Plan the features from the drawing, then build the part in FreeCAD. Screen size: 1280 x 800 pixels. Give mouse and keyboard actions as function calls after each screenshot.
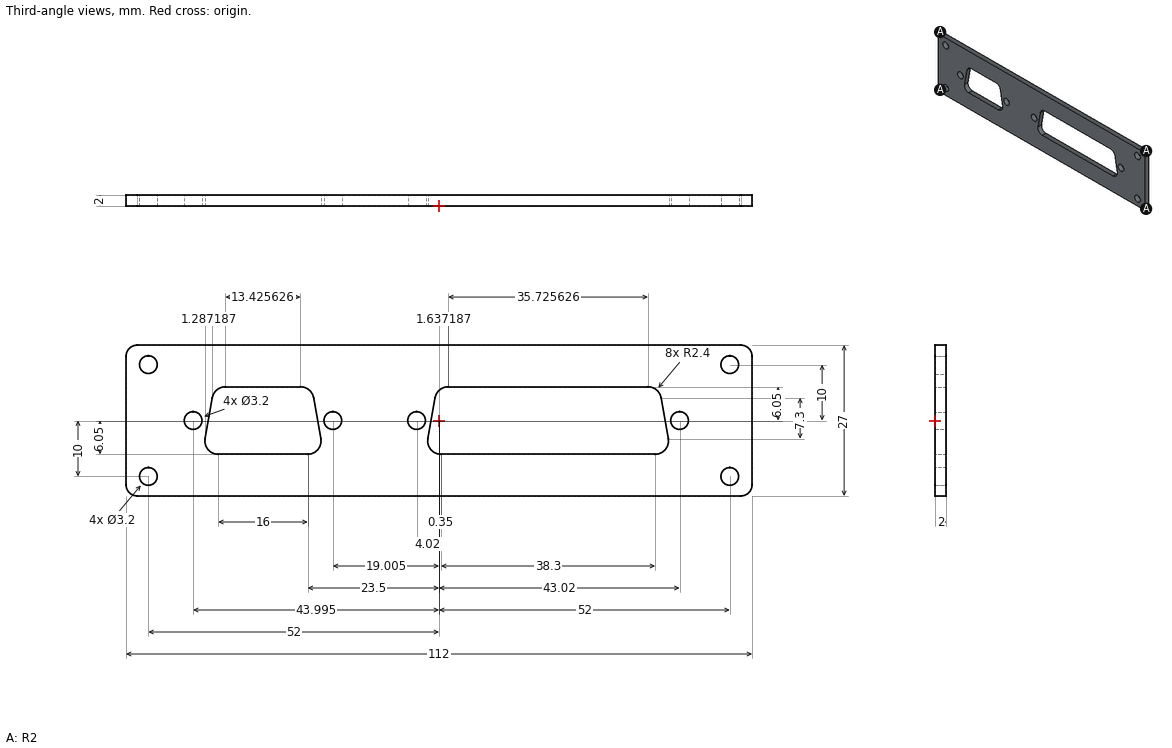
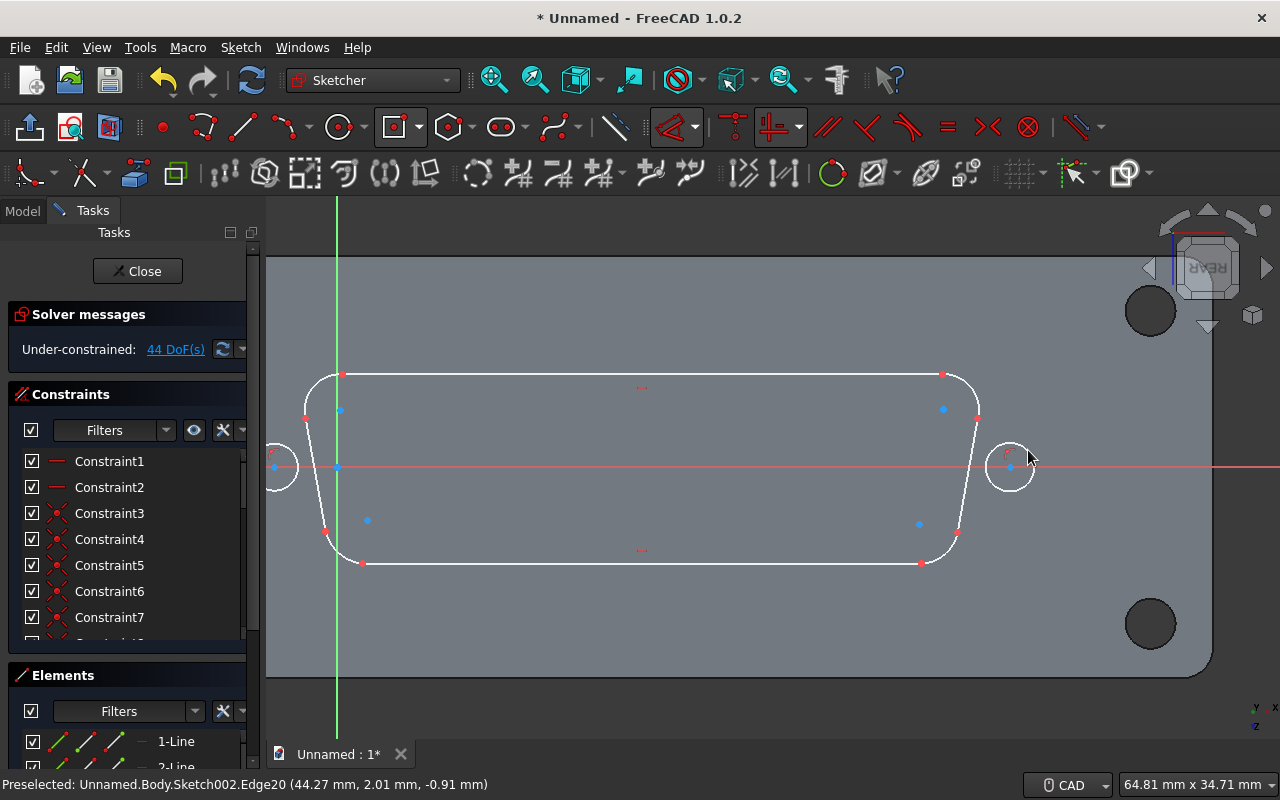
click(530, 564)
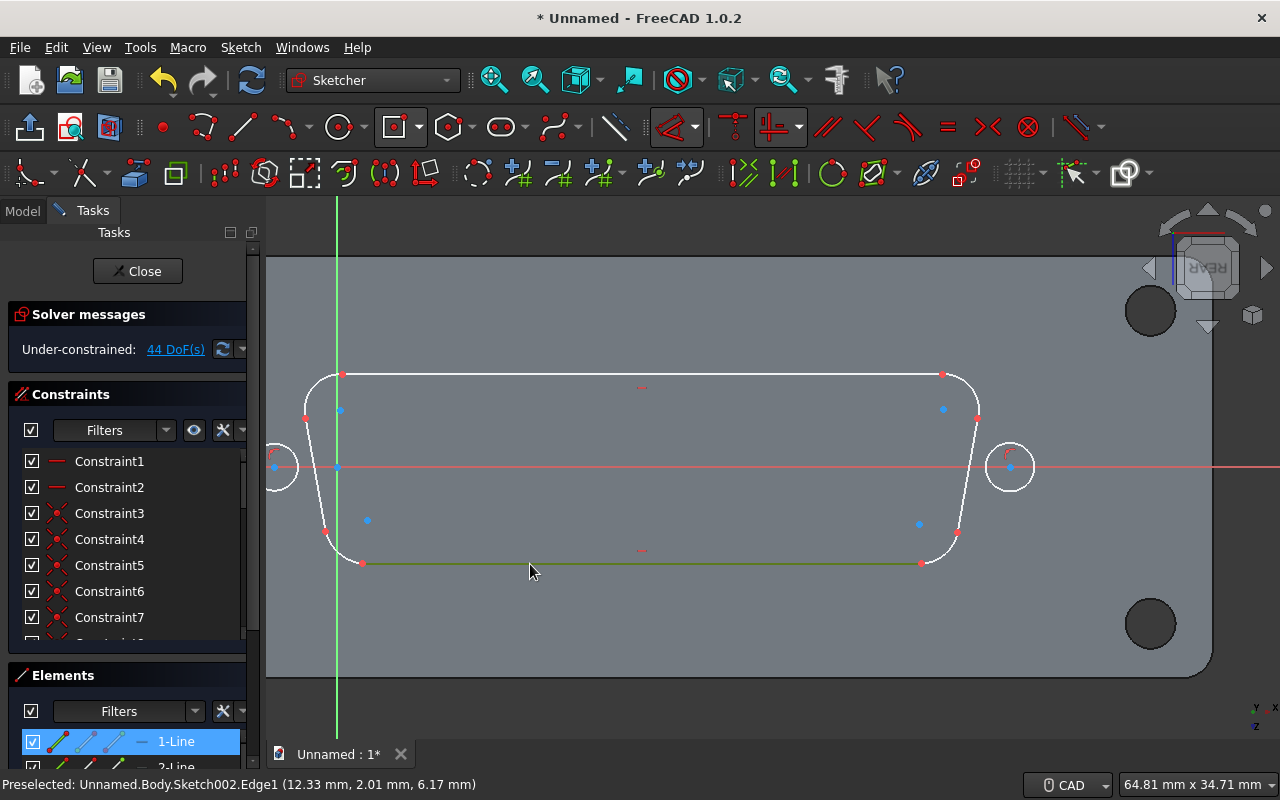
click(937, 560)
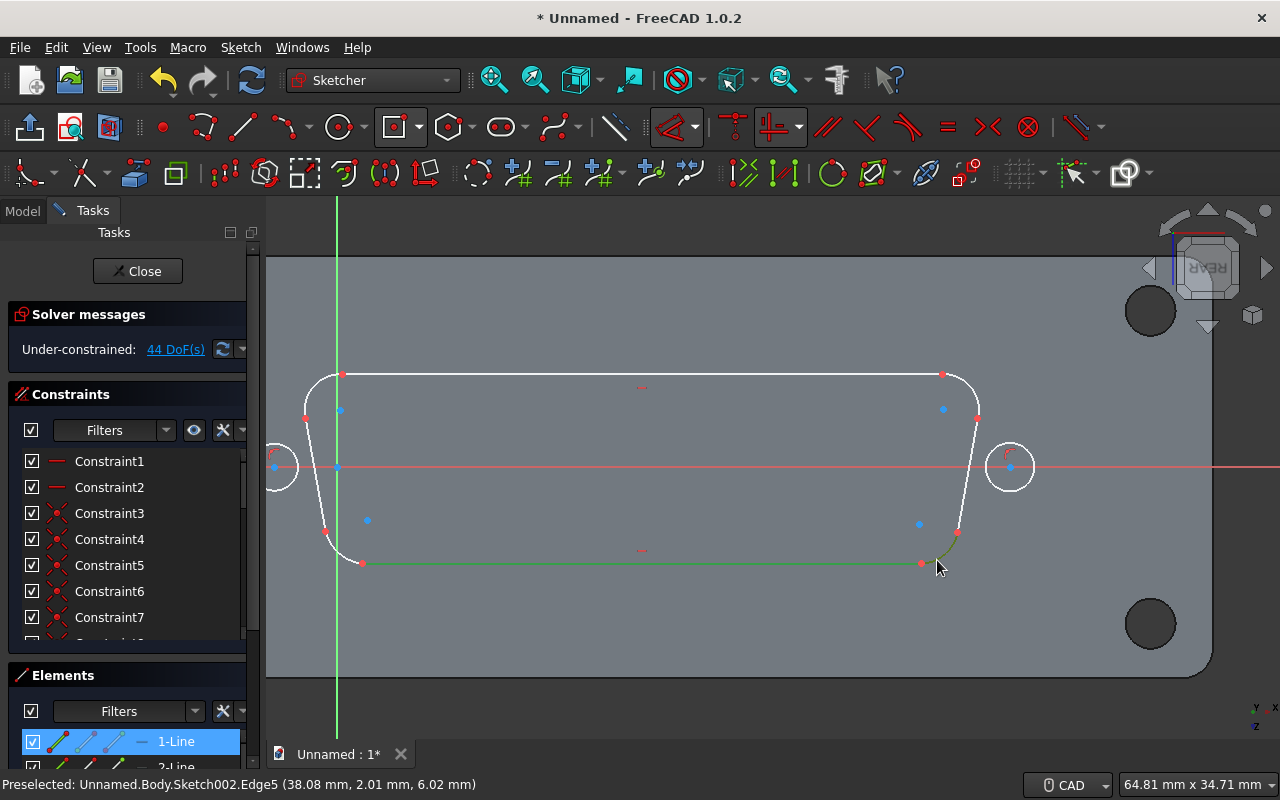
click(908, 128)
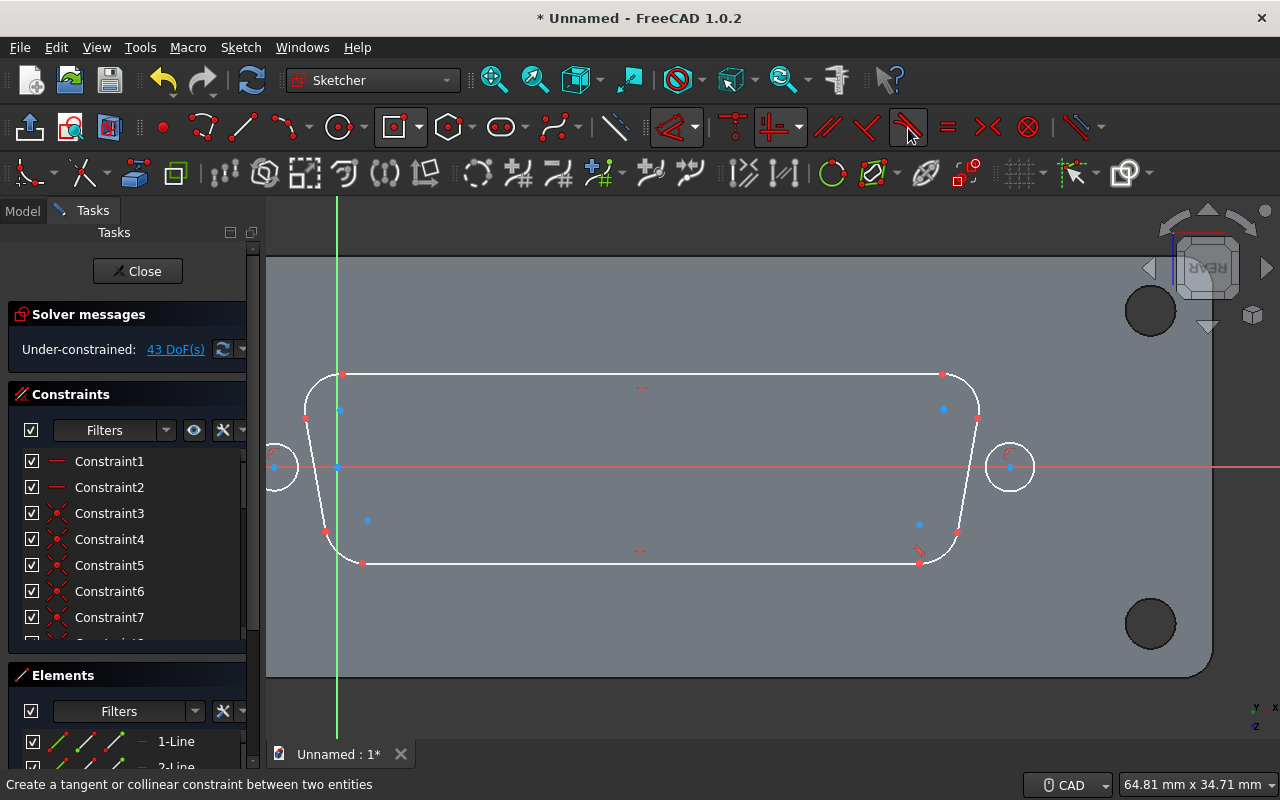
click(529, 564)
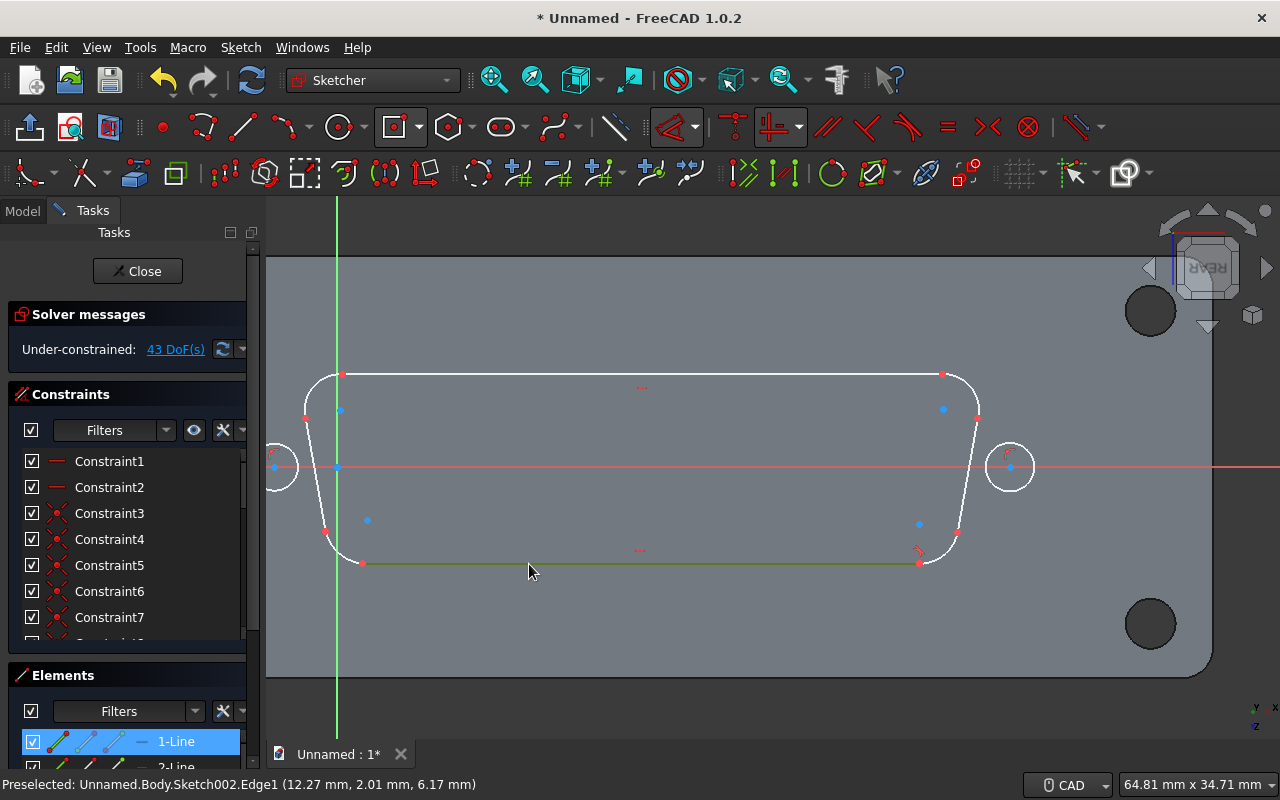
scroll(348, 559, up, 2)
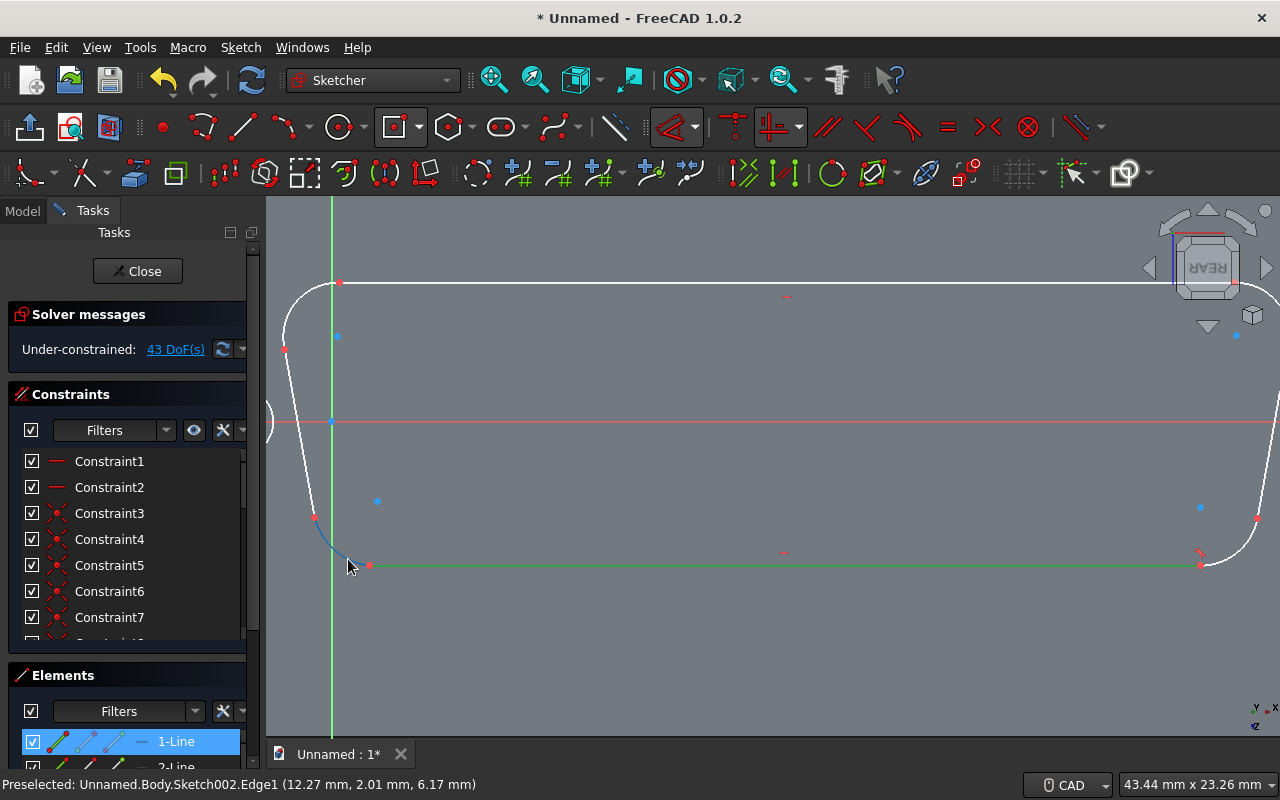
click(347, 559)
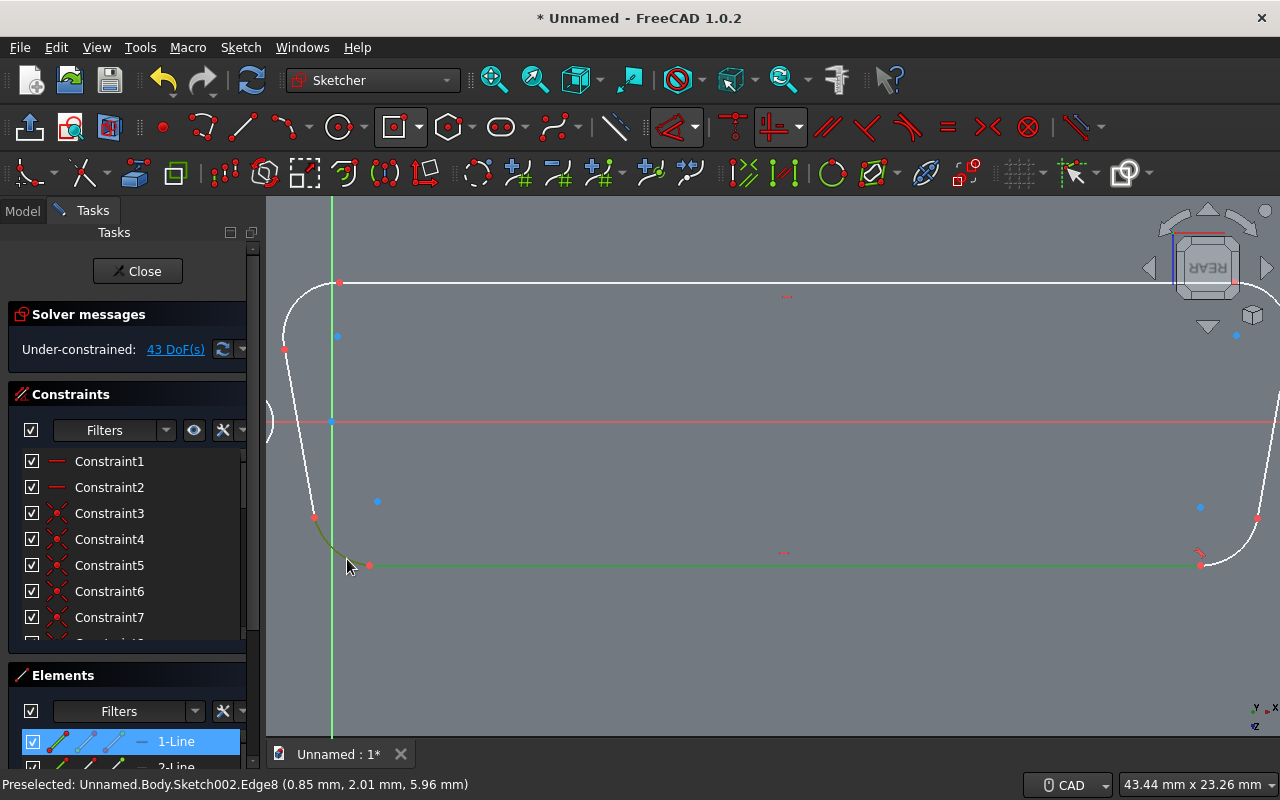
key(t)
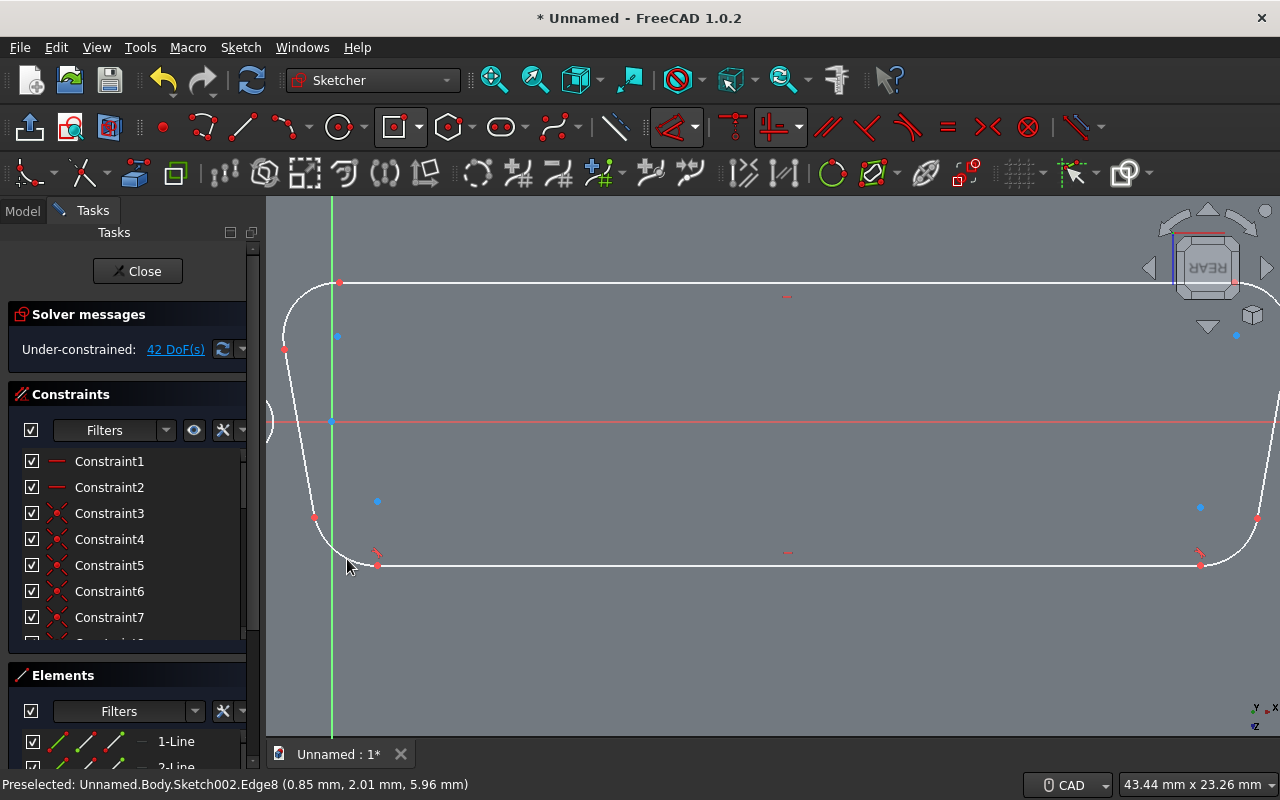
scroll(870, 487, down, 6)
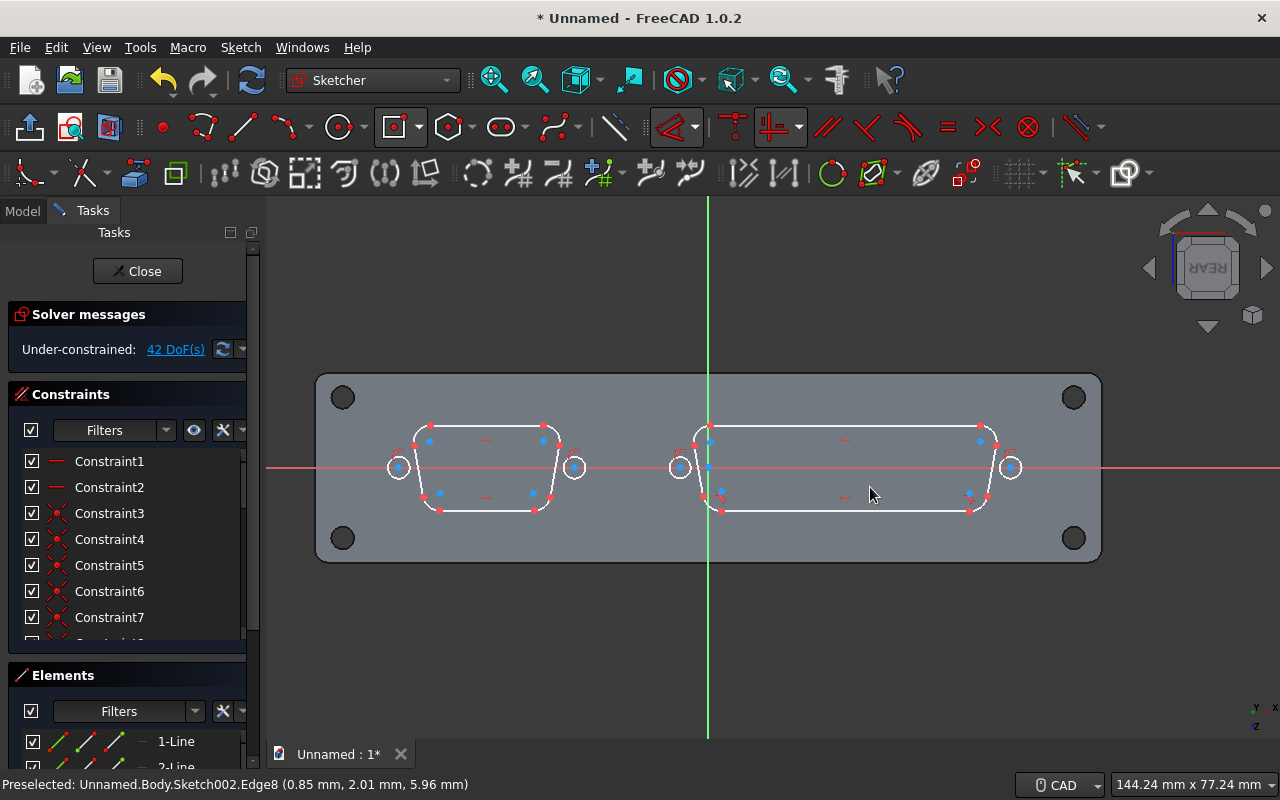
click(990, 482)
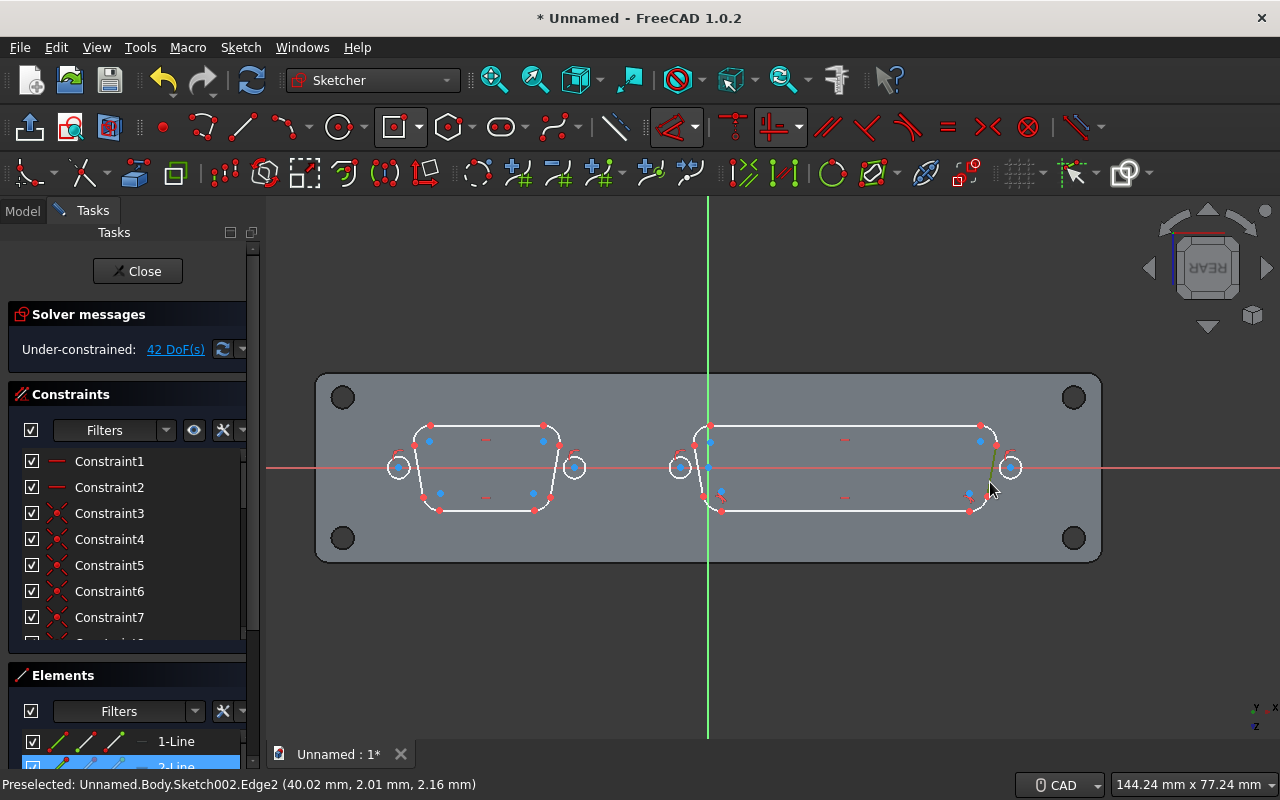
click(981, 507)